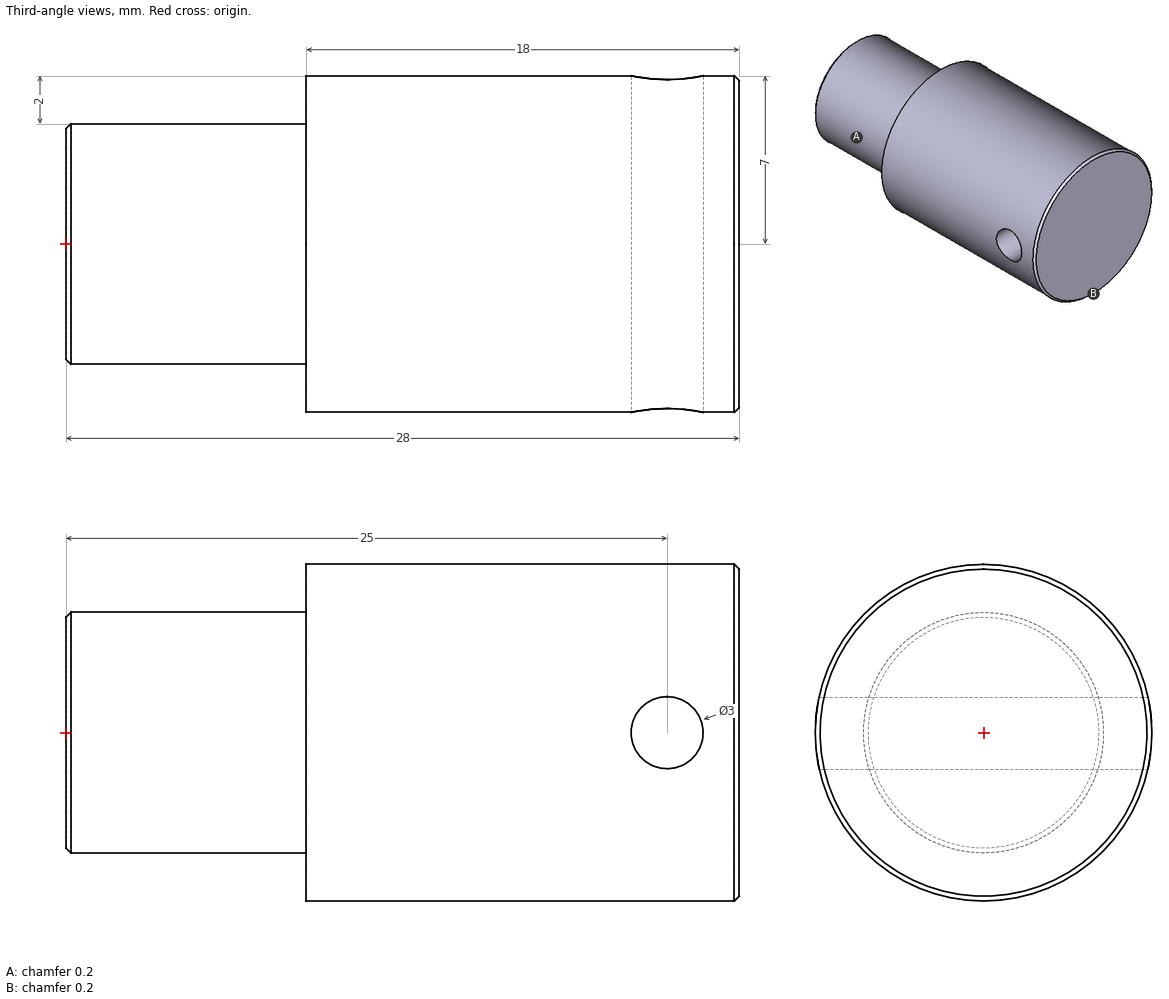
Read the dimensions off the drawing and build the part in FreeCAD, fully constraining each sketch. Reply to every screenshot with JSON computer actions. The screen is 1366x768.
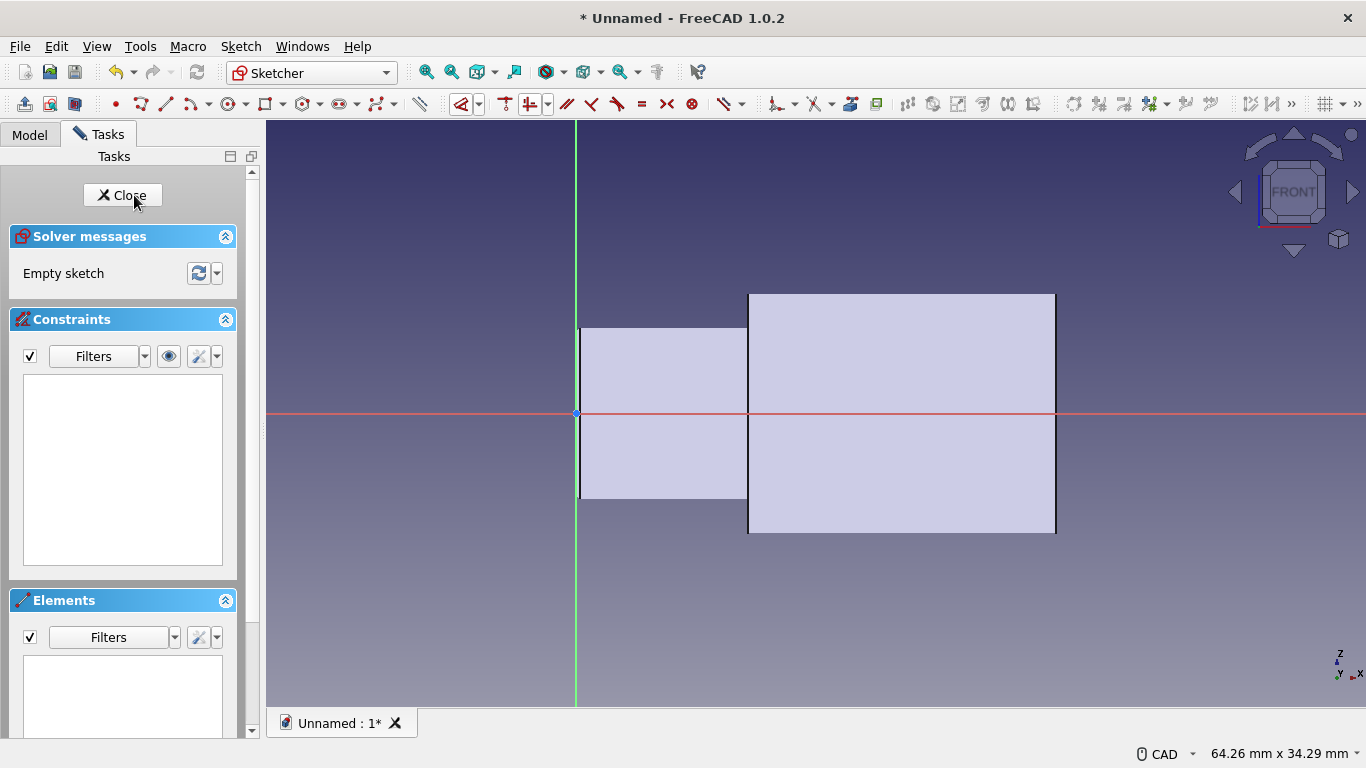
{"action": "scroll", "coordinate": [1044, 414], "scroll_direction": "up", "scroll_amount": 10}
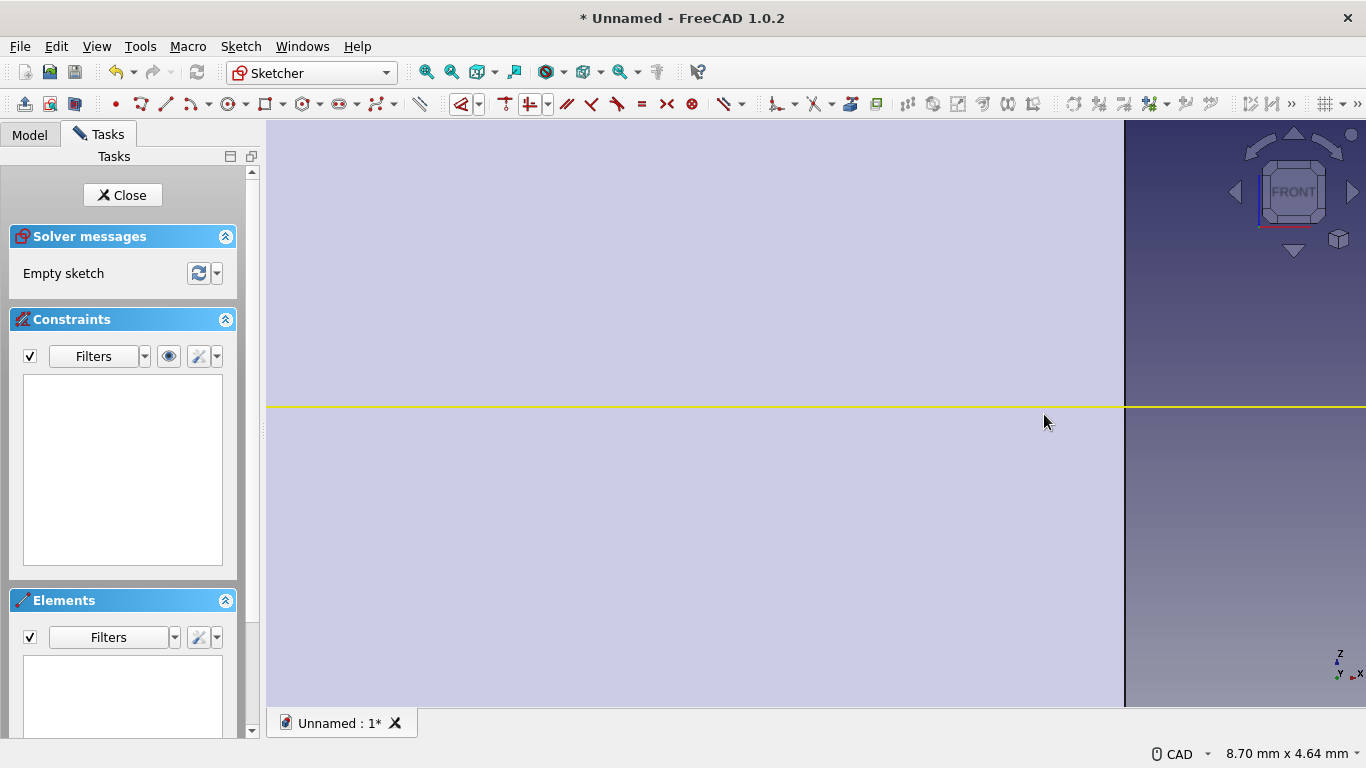
{"action": "key", "text": "g c"}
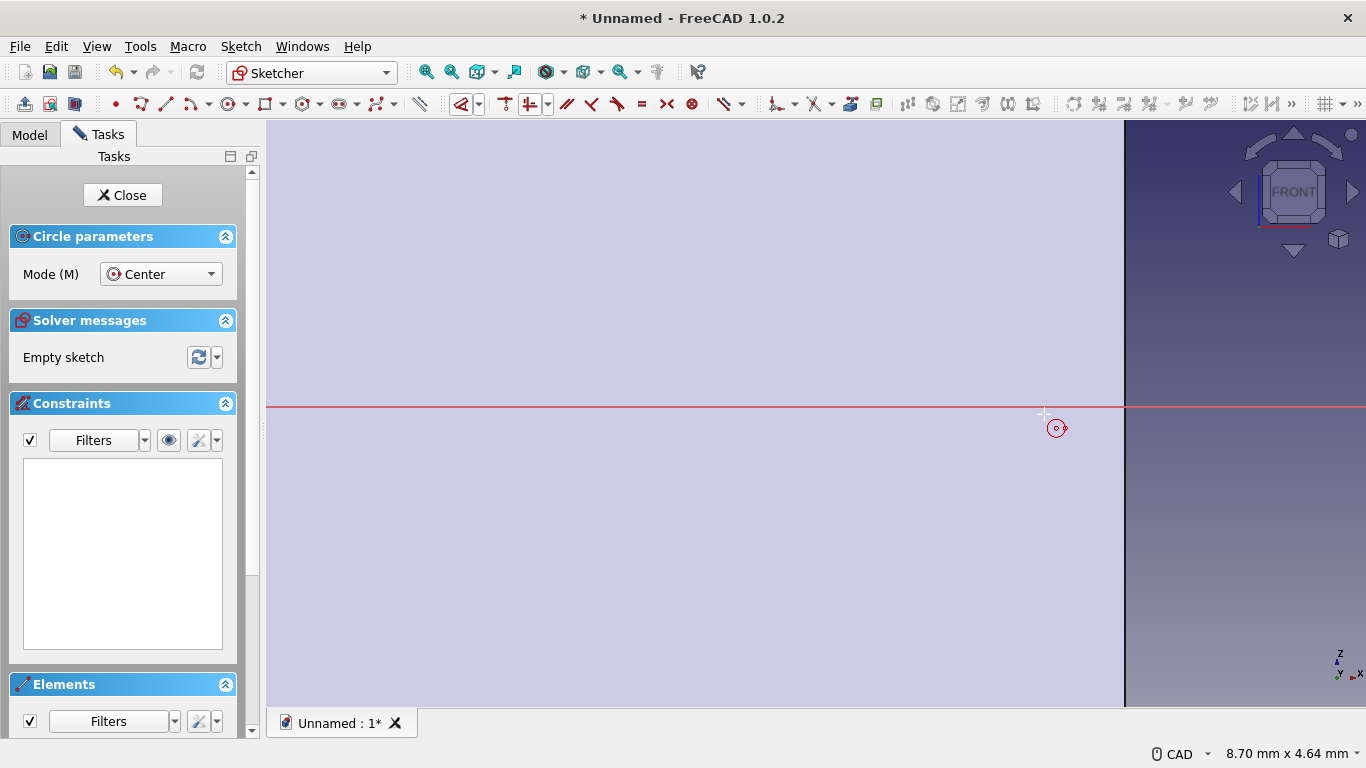
{"action": "left_click", "coordinate": [746, 407]}
{"action": "left_click", "coordinate": [880, 273]}
{"action": "key", "text": "Escape"}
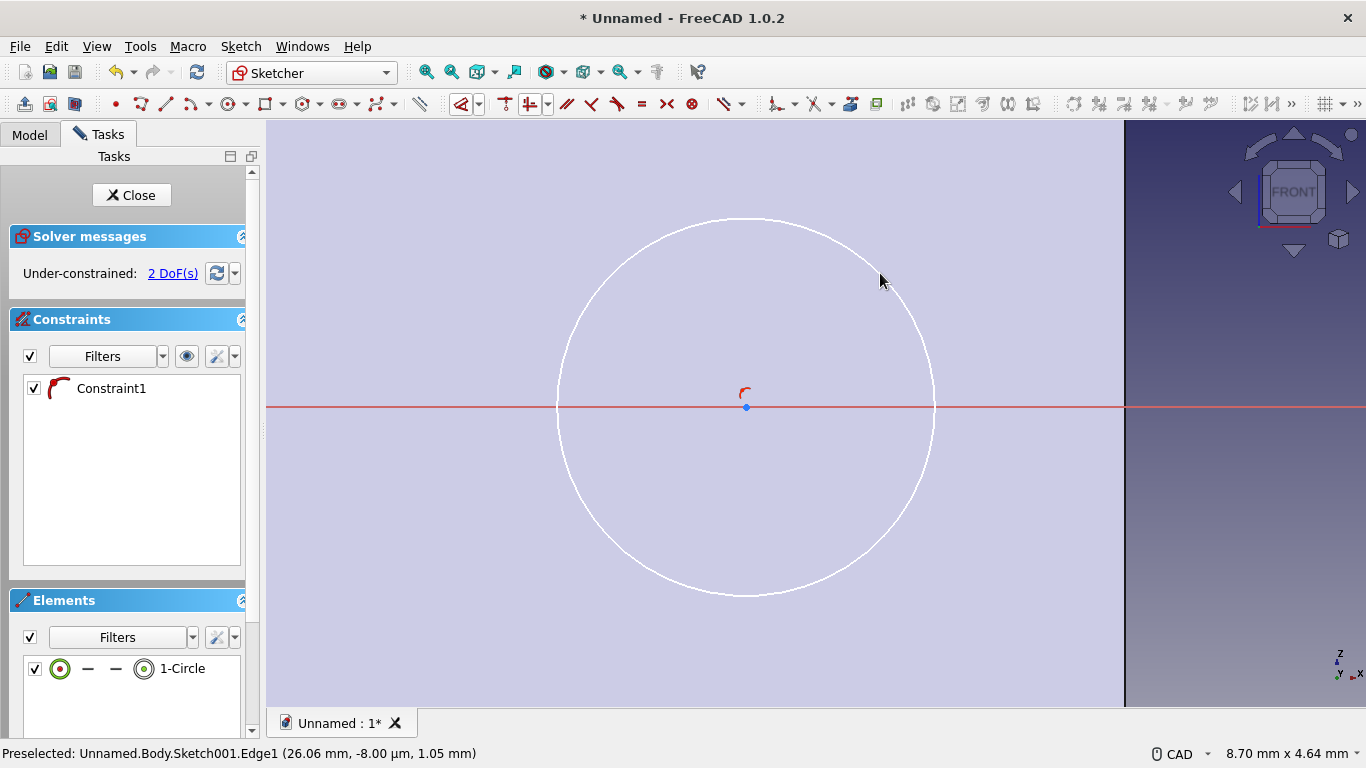
{"action": "key", "text": "d"}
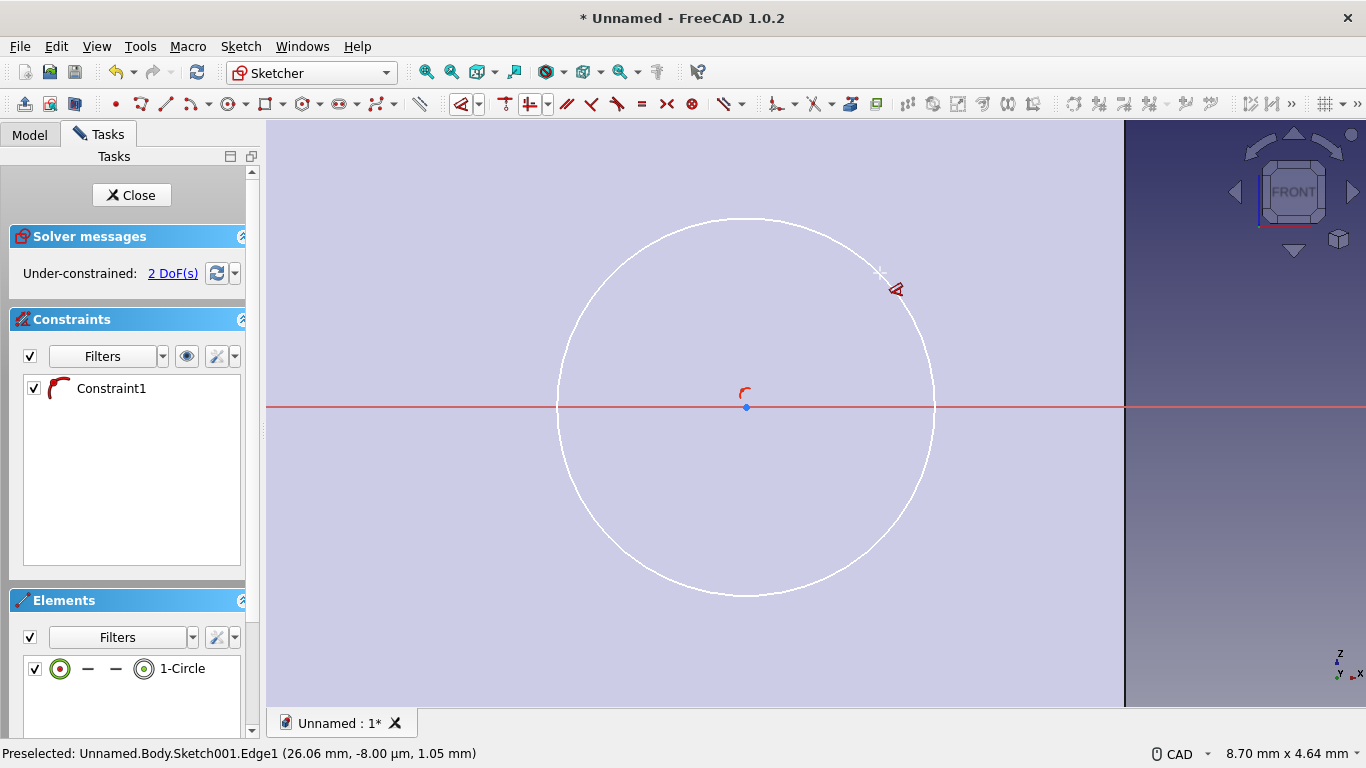
{"action": "left_click", "coordinate": [879, 273]}
{"action": "left_click", "coordinate": [902, 250]}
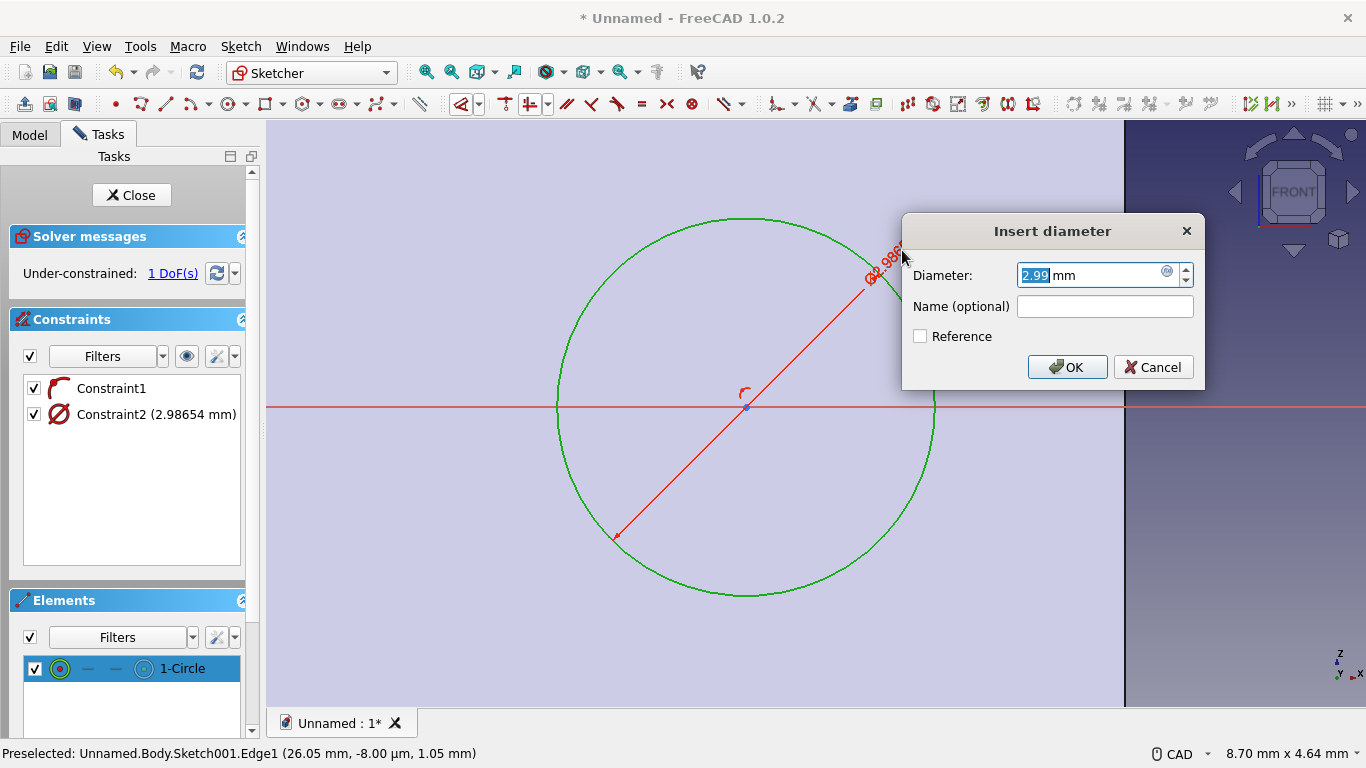
{"action": "type", "text": "3"}
{"action": "key", "text": "Return"}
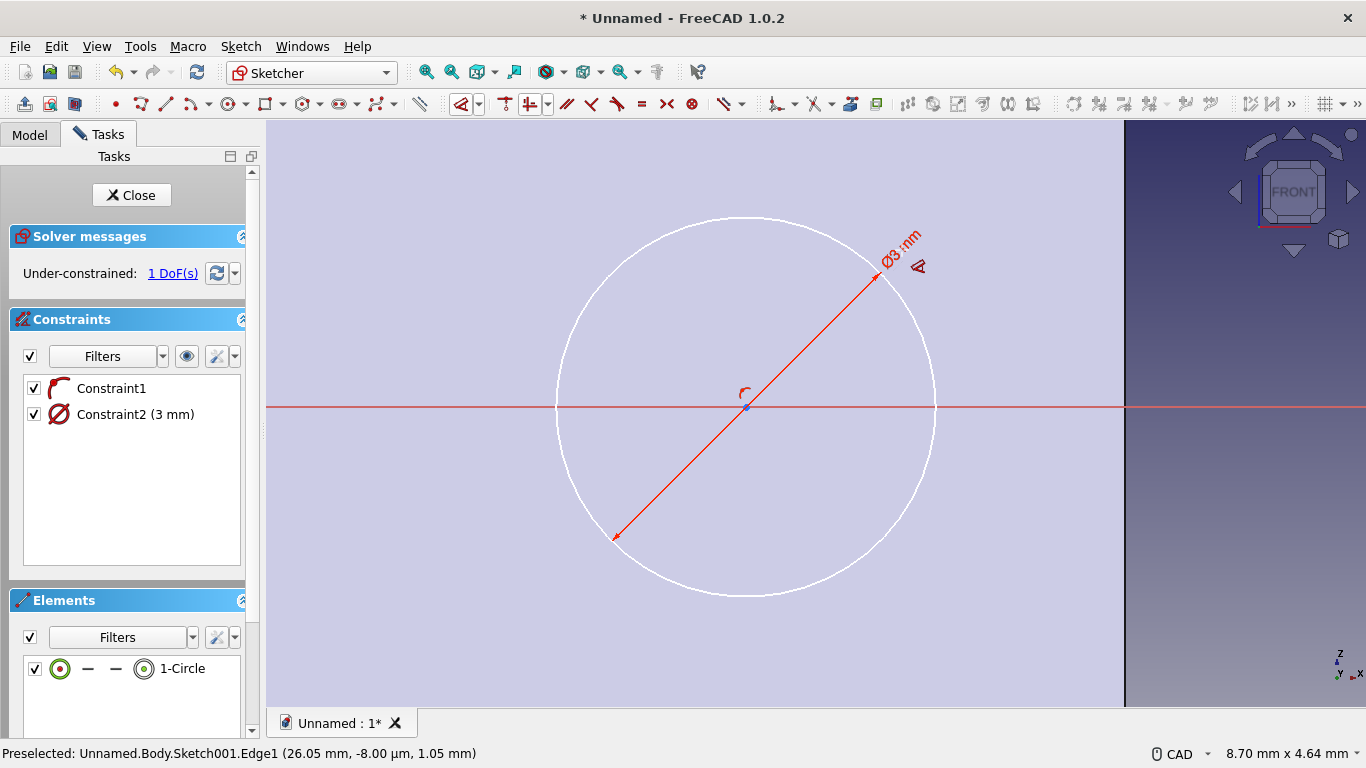
{"action": "left_click", "coordinate": [746, 407]}
{"action": "left_click", "coordinate": [520, 441]}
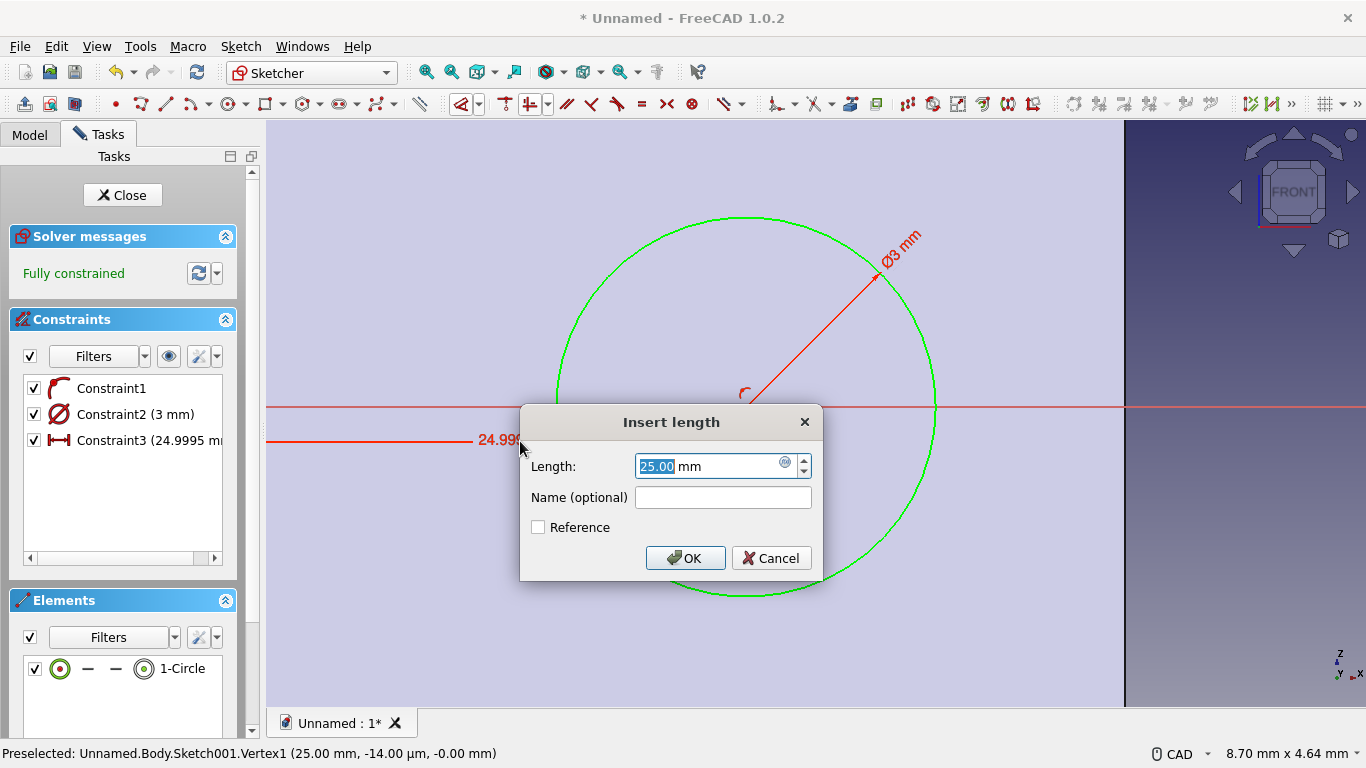
{"action": "type", "text": "25"}
{"action": "key", "text": "Return"}
{"action": "key", "text": "Escape"}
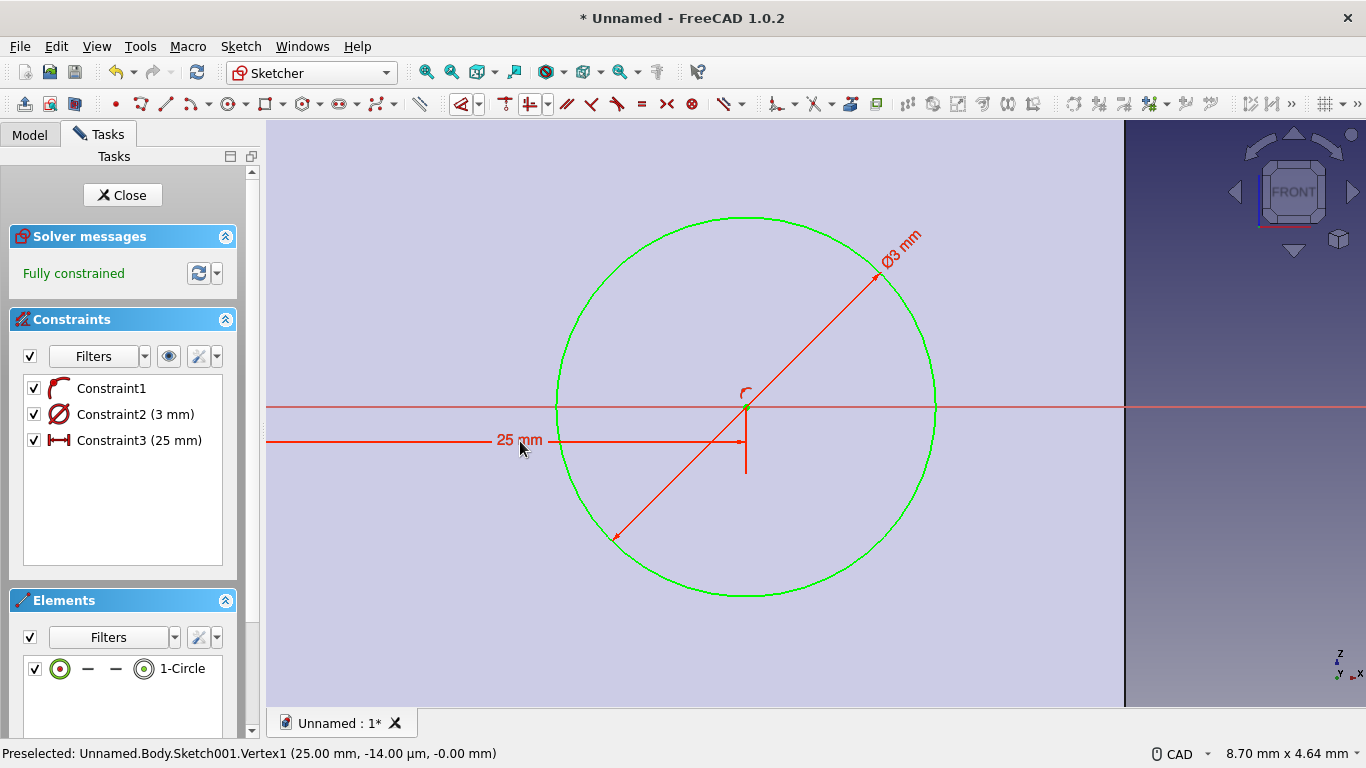
{"action": "left_click", "coordinate": [123, 195]}